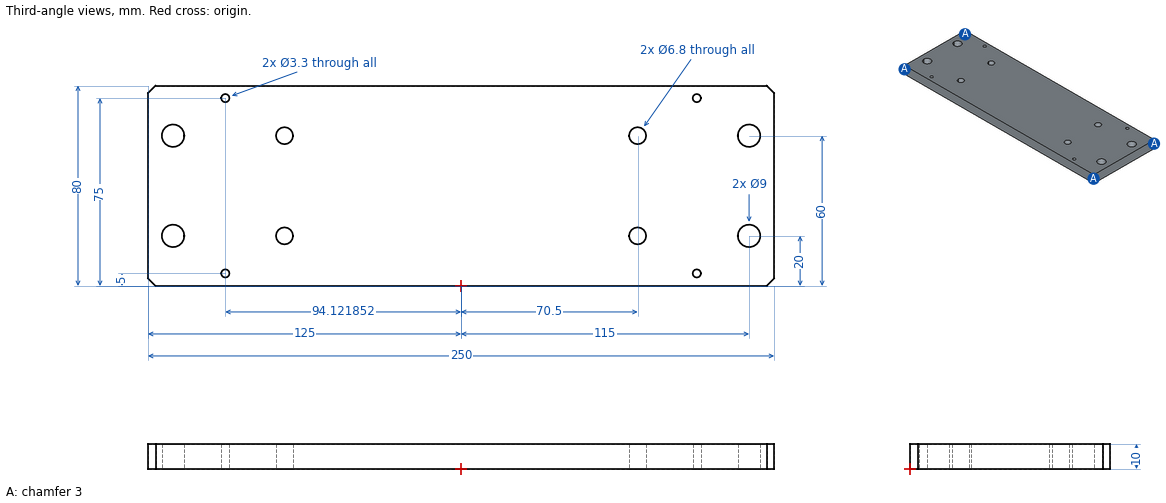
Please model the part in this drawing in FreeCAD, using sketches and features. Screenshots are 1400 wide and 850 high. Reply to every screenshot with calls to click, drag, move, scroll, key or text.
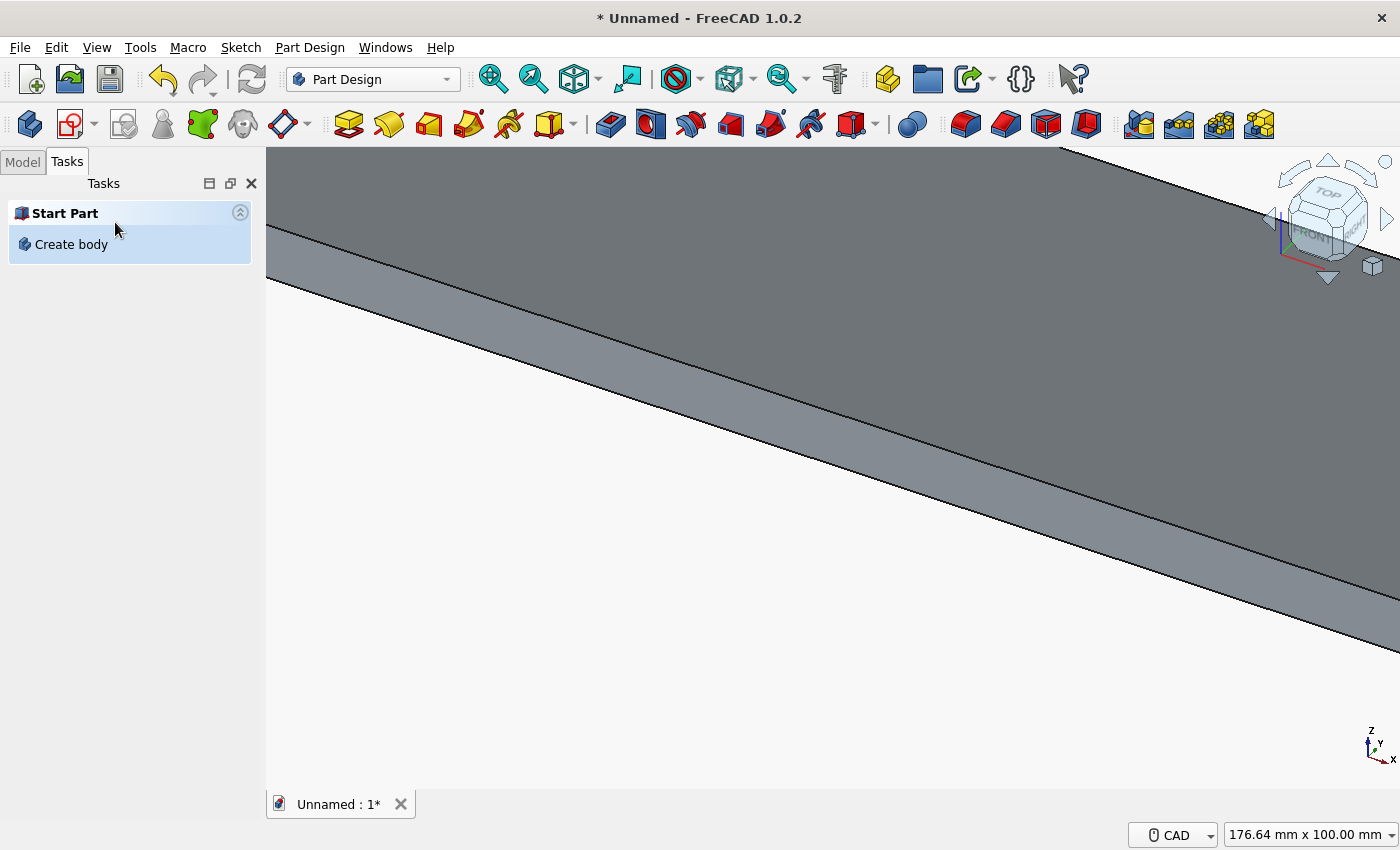
click(494, 80)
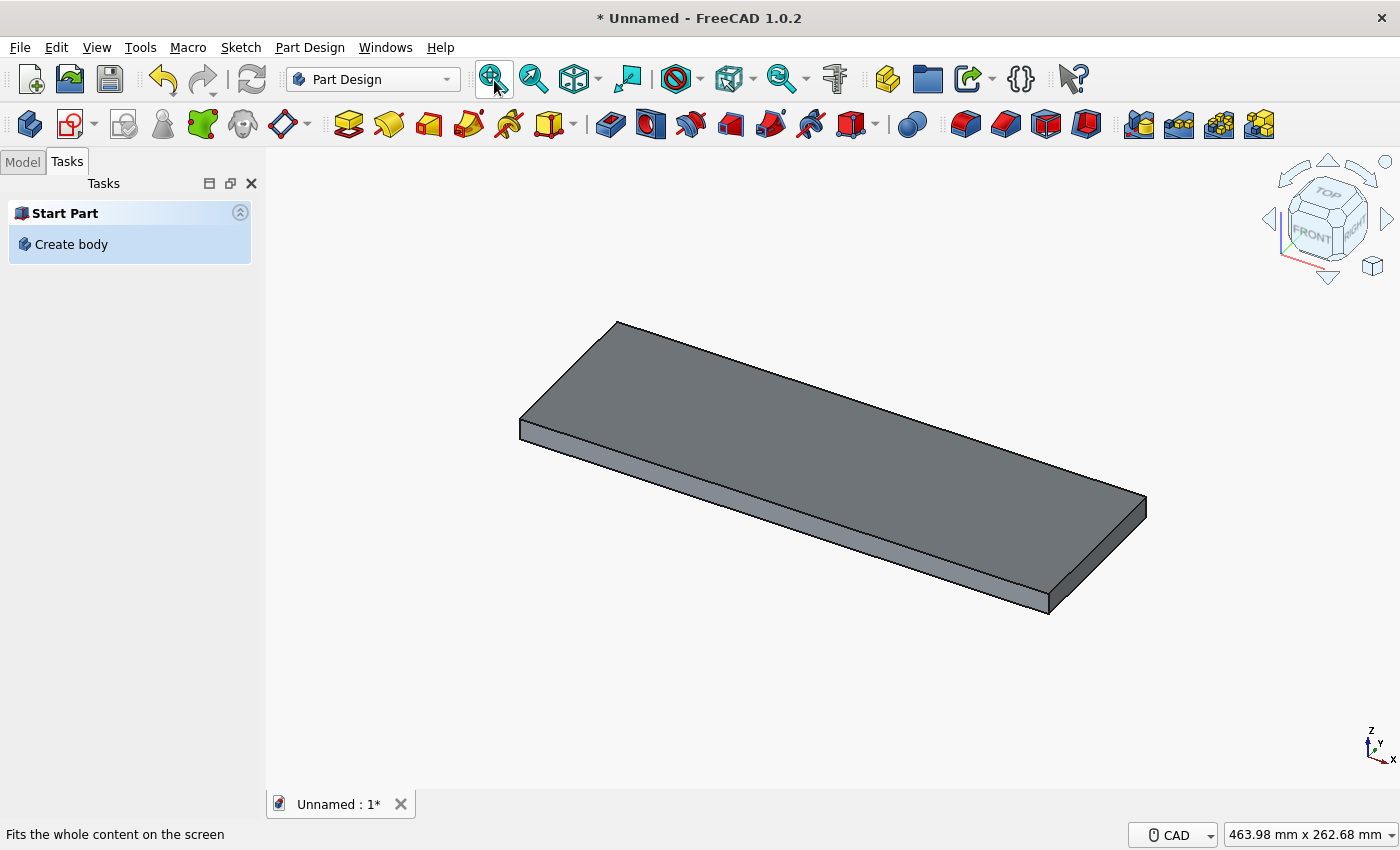
click(984, 507)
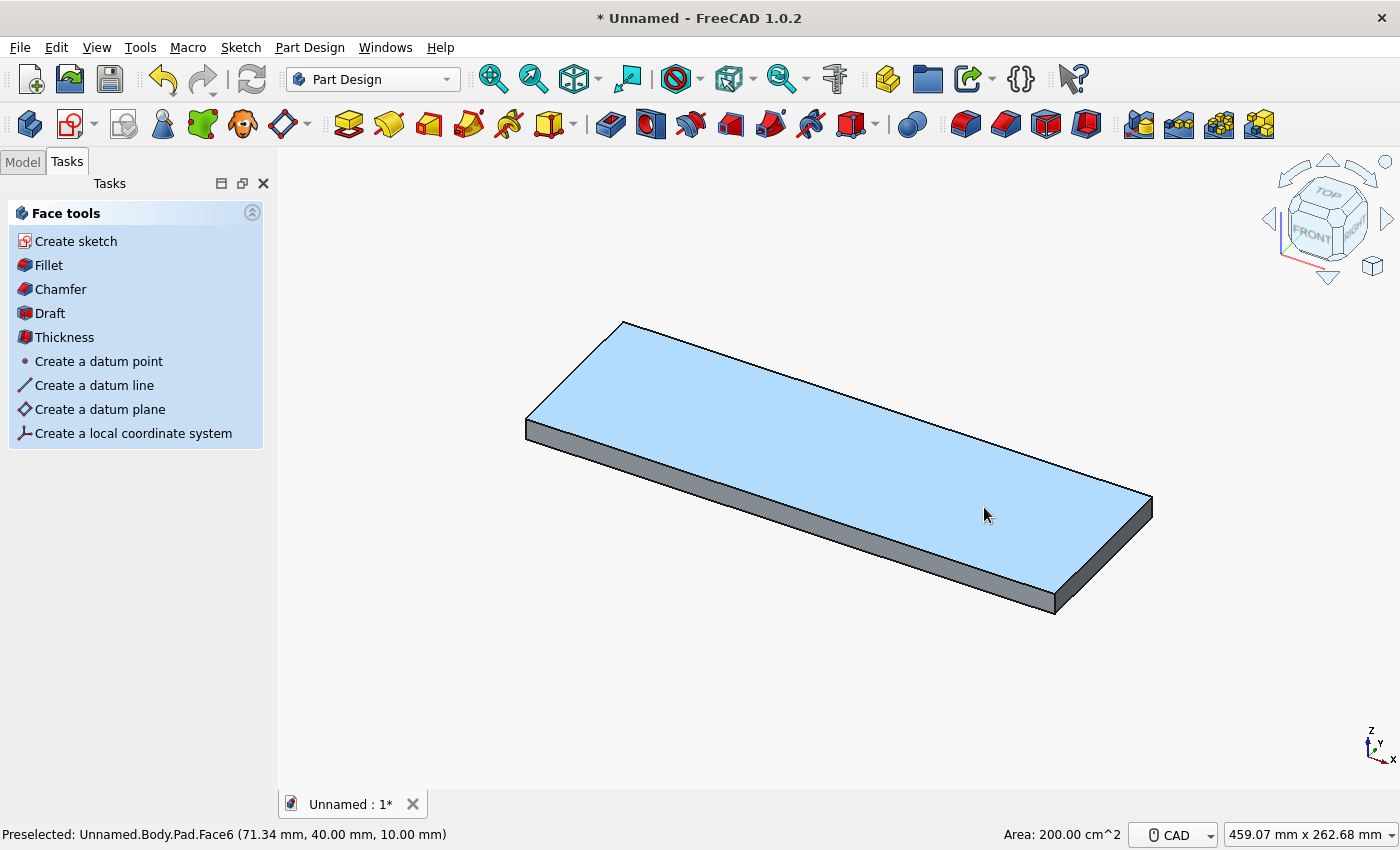
click(70, 124)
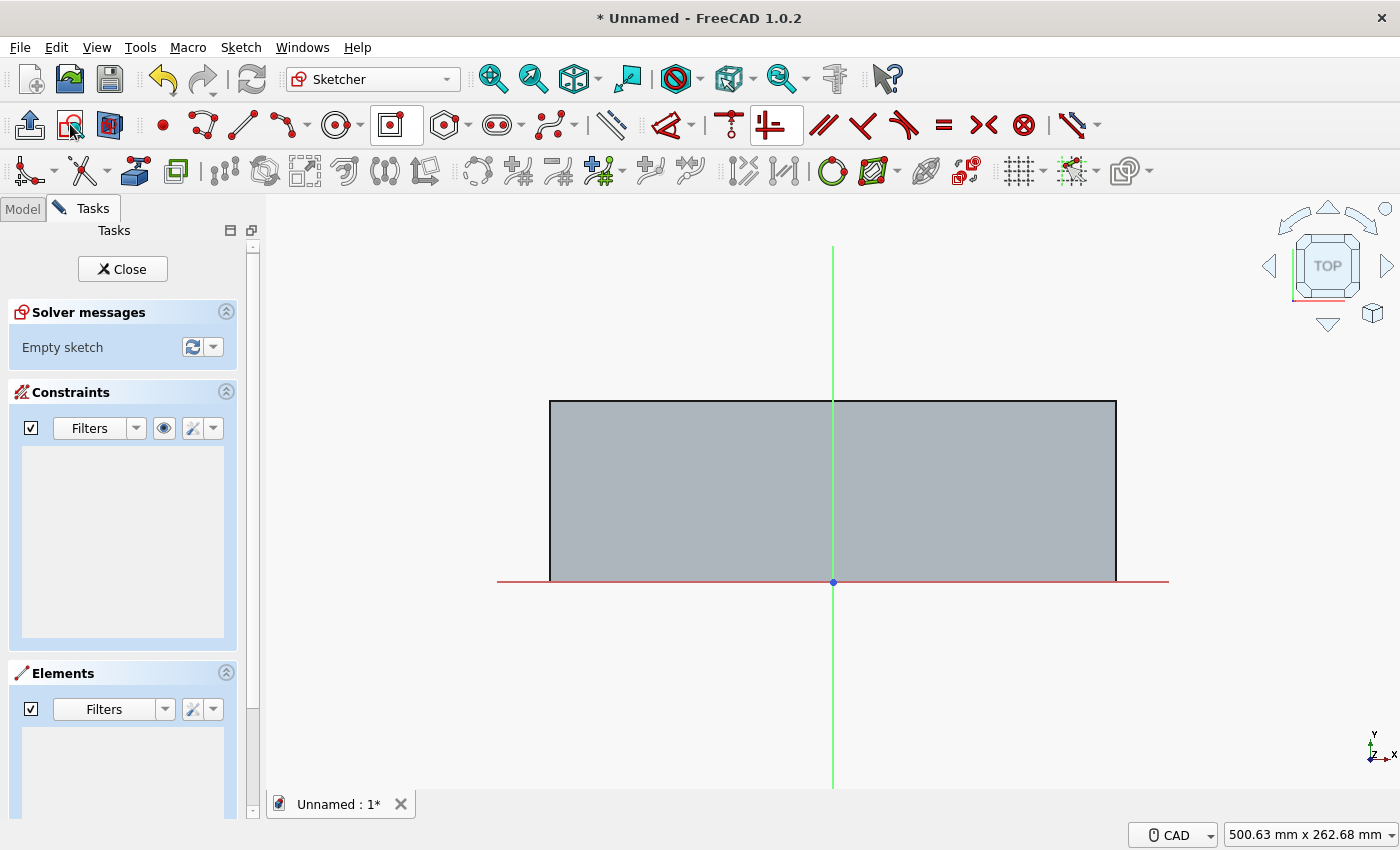
scroll(1135, 523, up, 4)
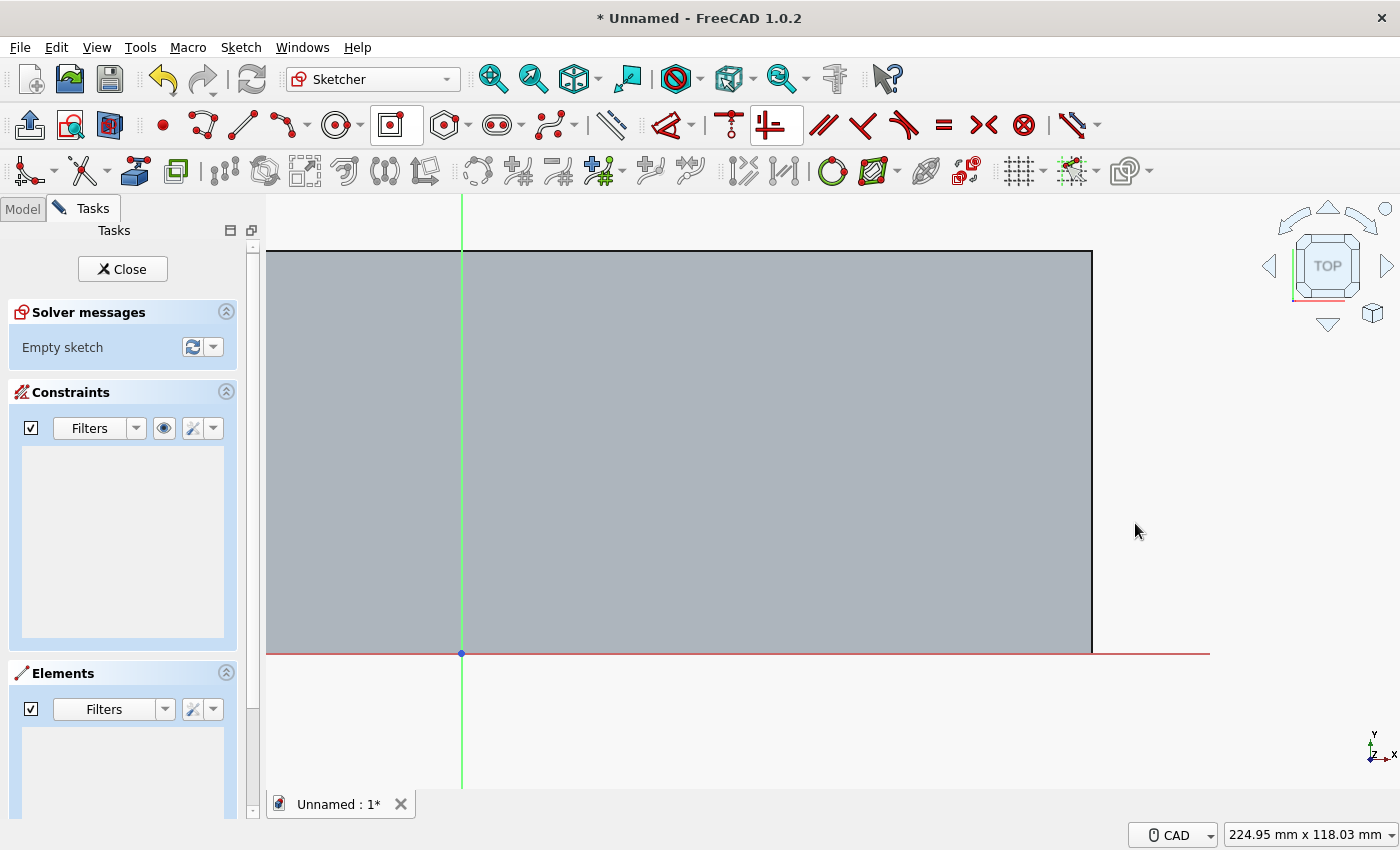
click(336, 126)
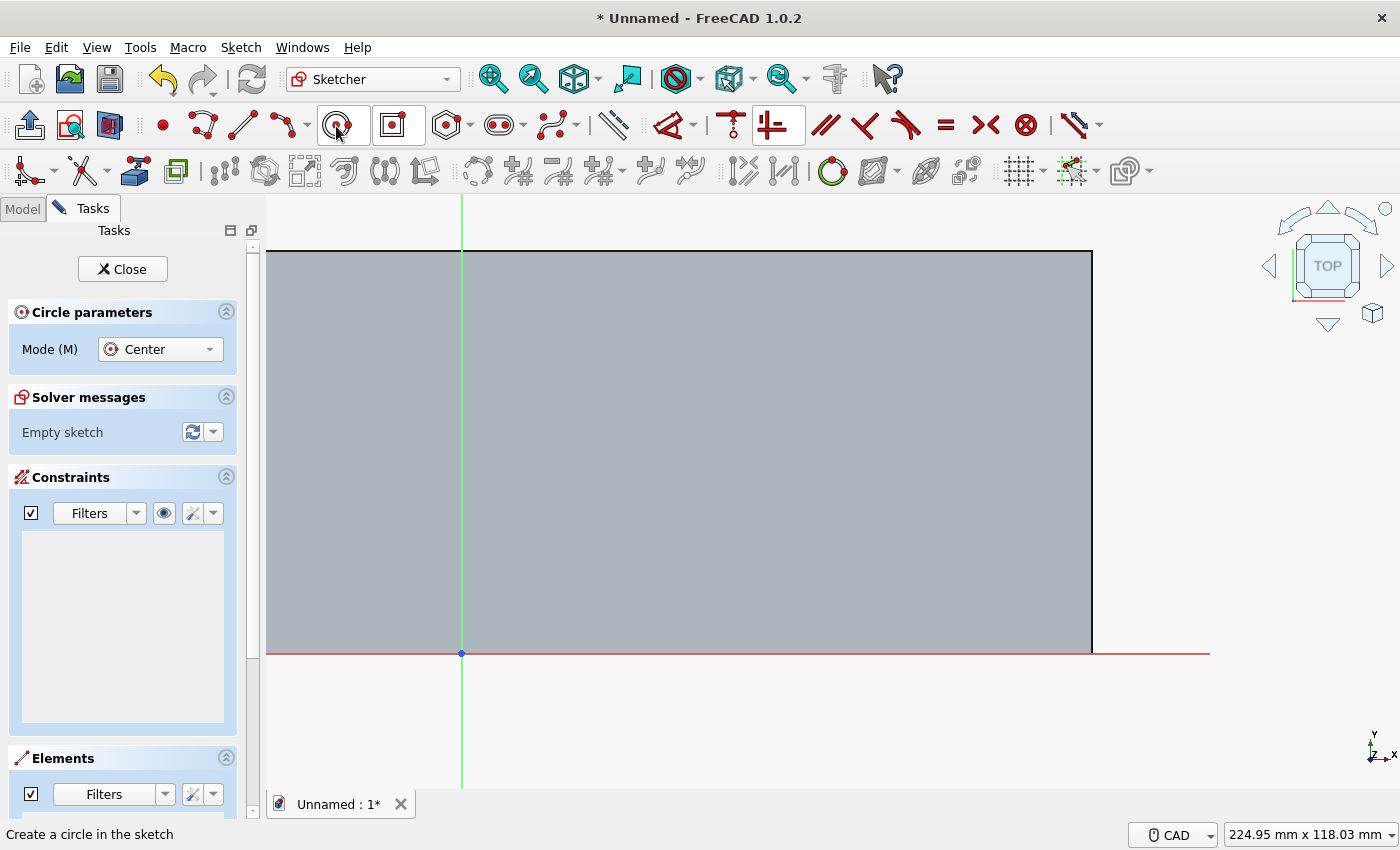
click(1042, 553)
move(1058, 537)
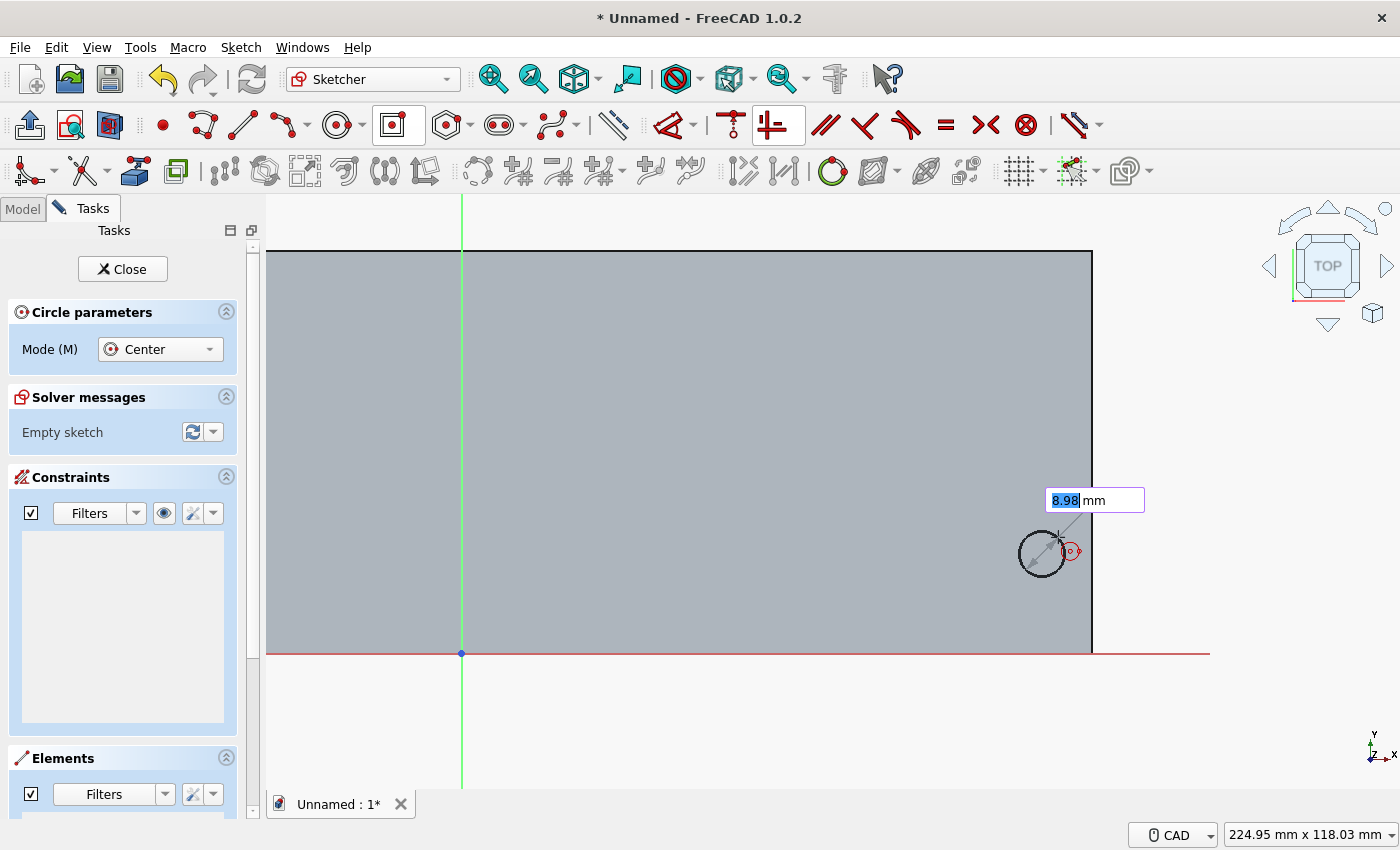
text(9)
key(Return)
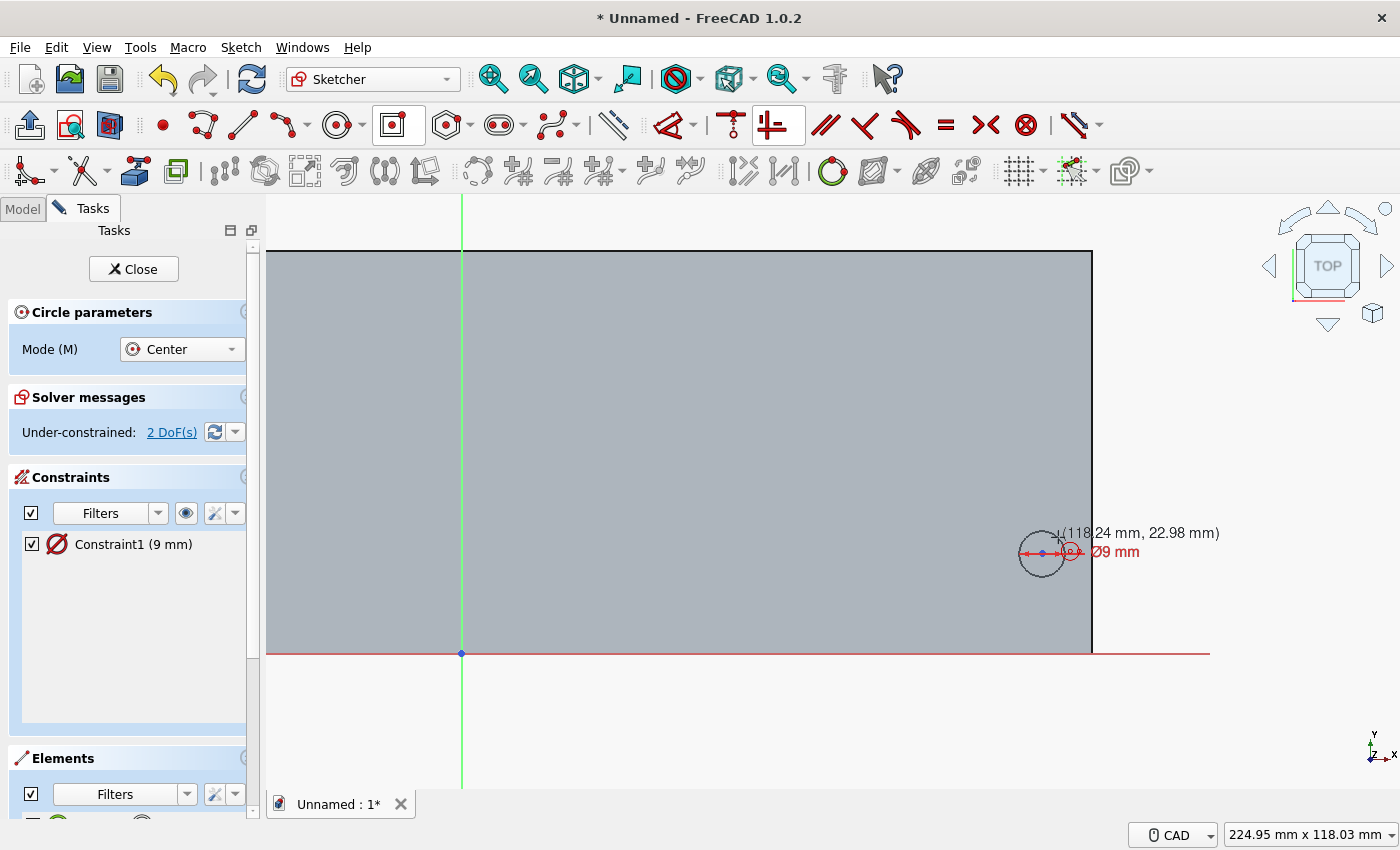
click(1042, 351)
move(1058, 335)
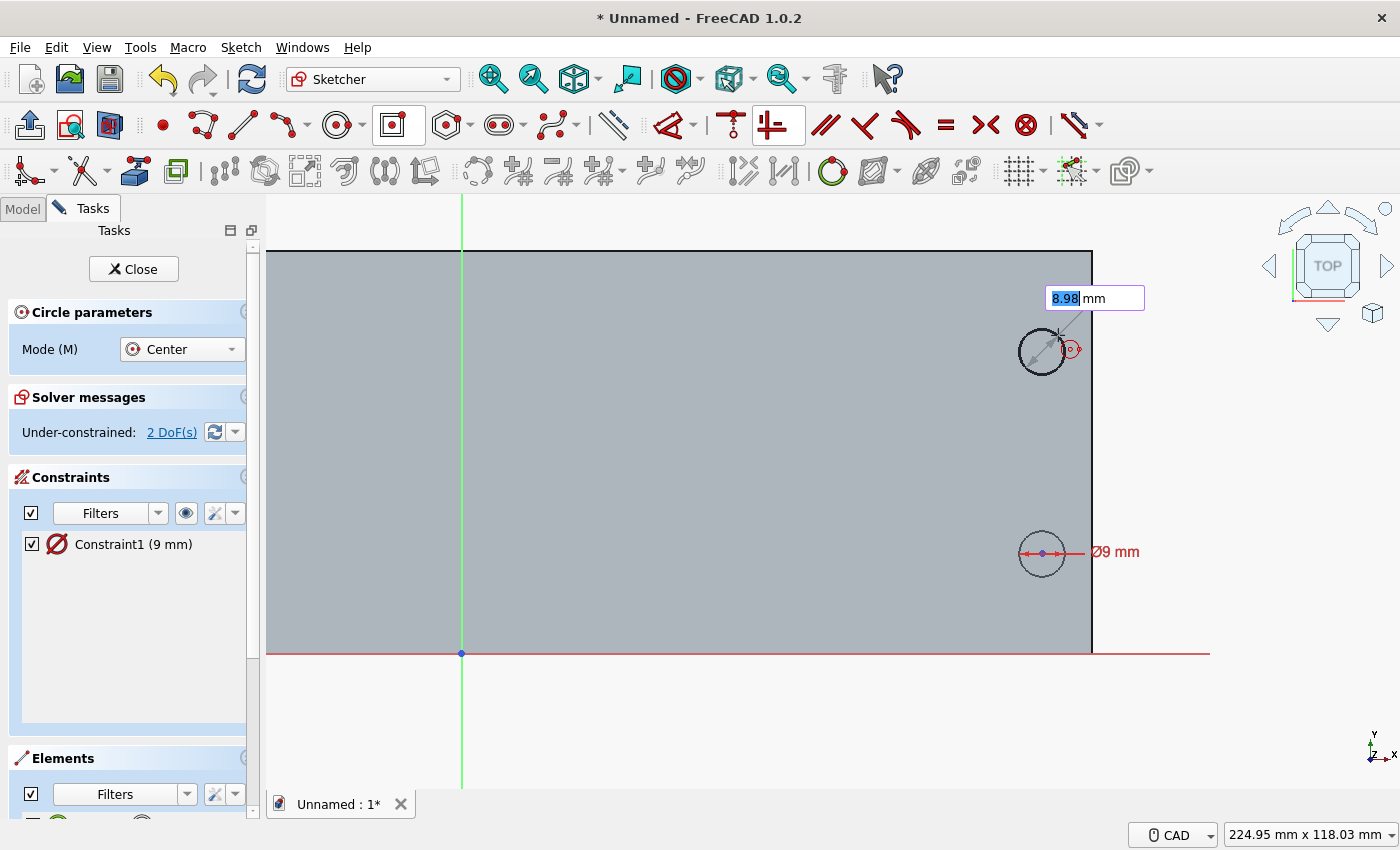
text(9)
key(Return)
key(Escape)